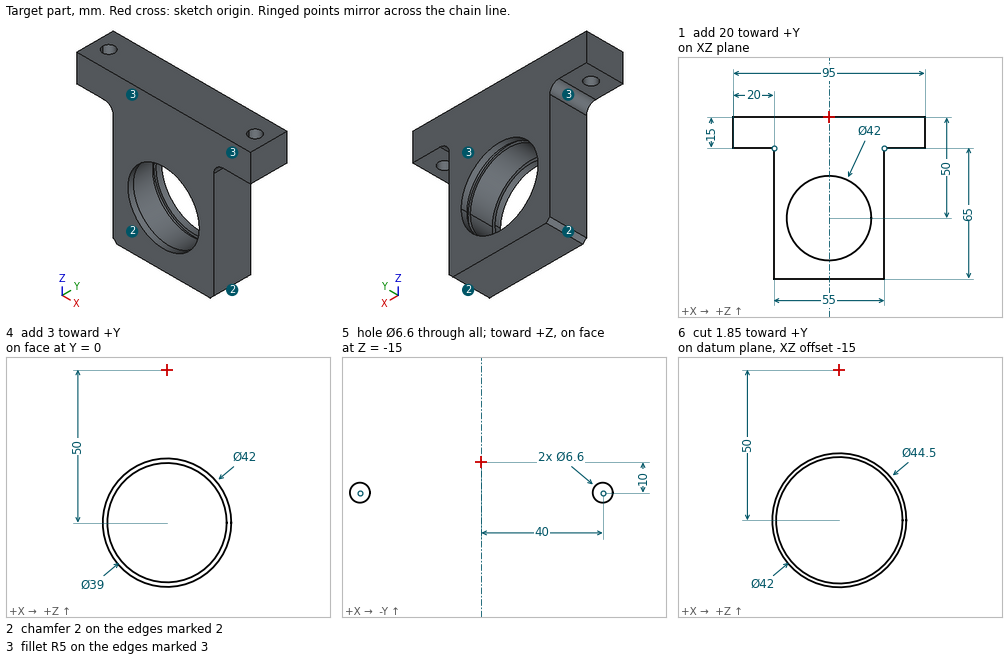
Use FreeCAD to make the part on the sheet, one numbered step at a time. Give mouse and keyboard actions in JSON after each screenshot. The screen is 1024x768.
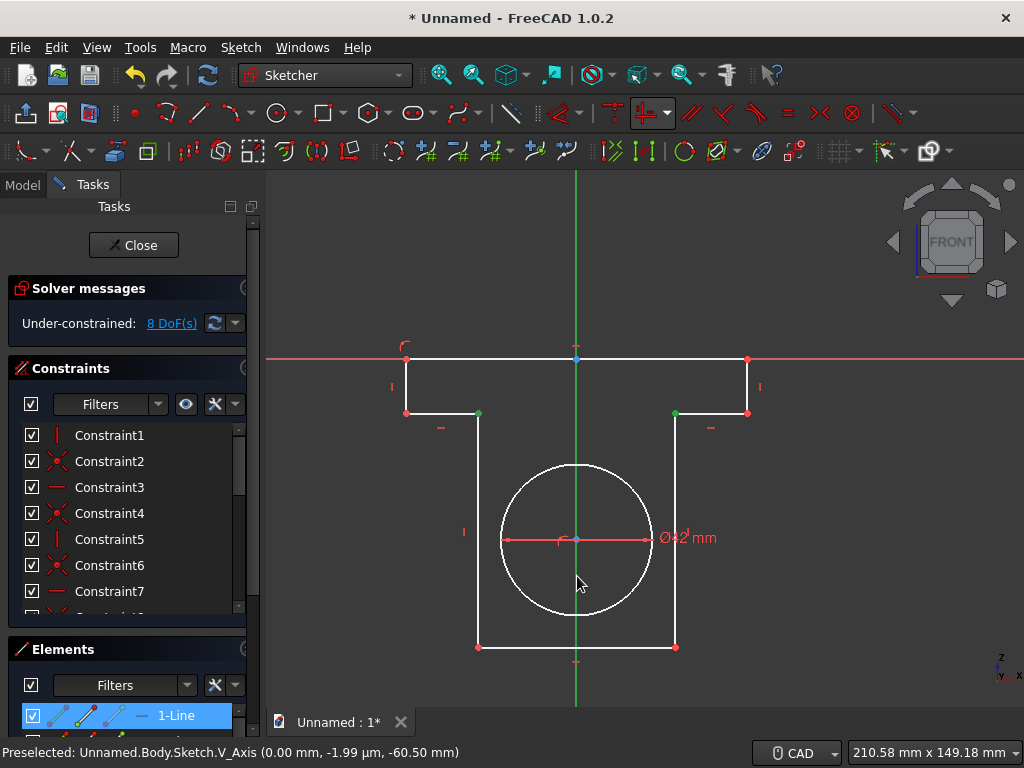
{"action": "left_click", "coordinate": [820, 114]}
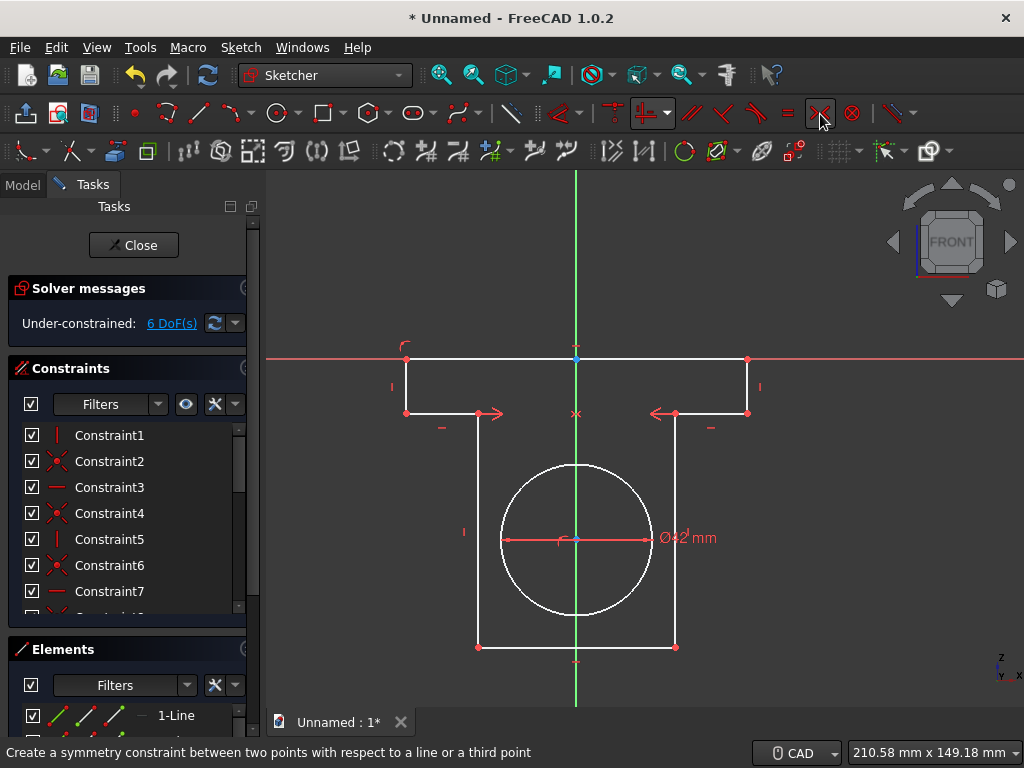
{"action": "left_click", "coordinate": [675, 484]}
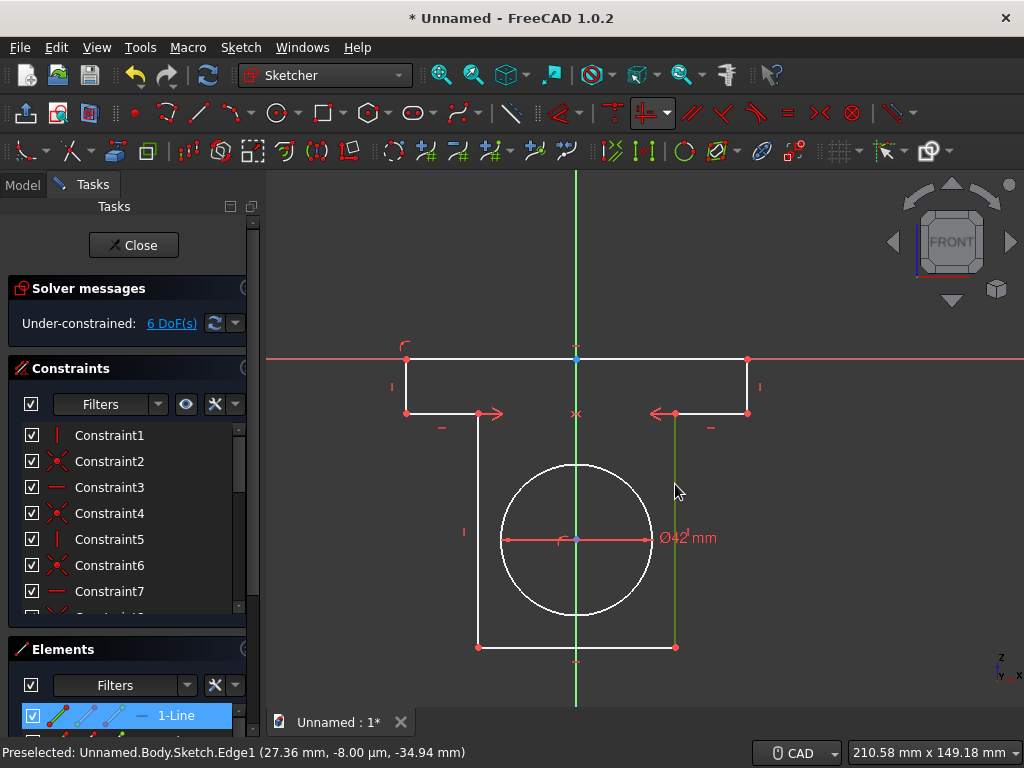
{"action": "key", "text": "i"}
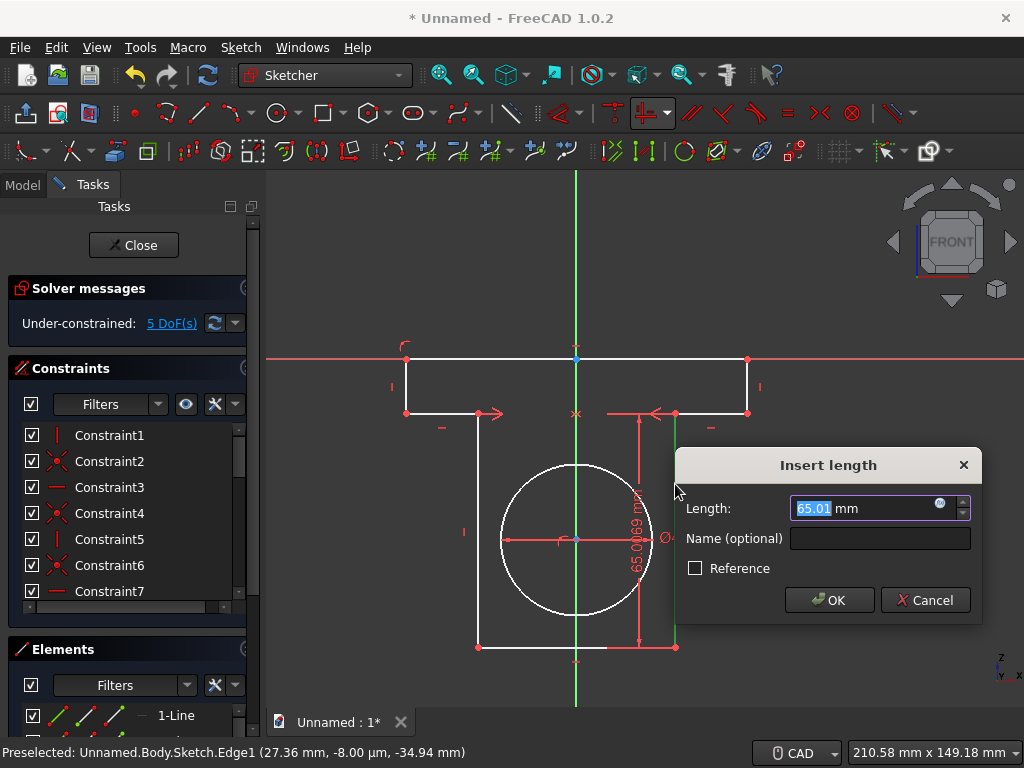
{"action": "type", "text": "65"}
{"action": "key", "text": "Return"}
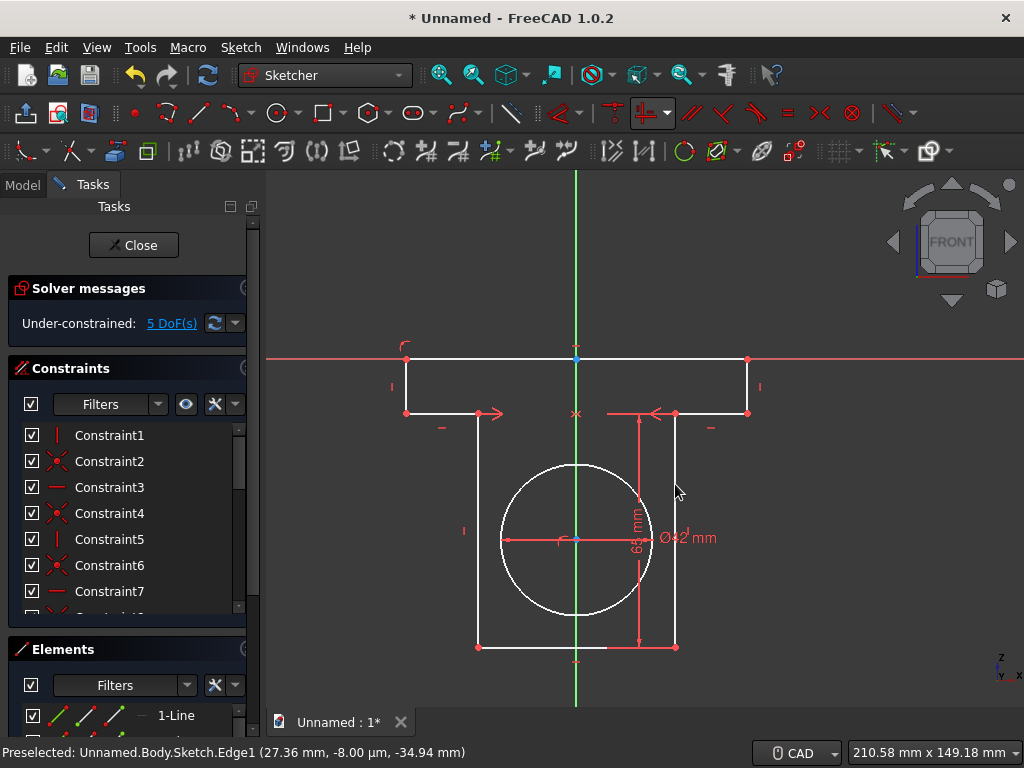
{"action": "left_click", "coordinate": [616, 648]}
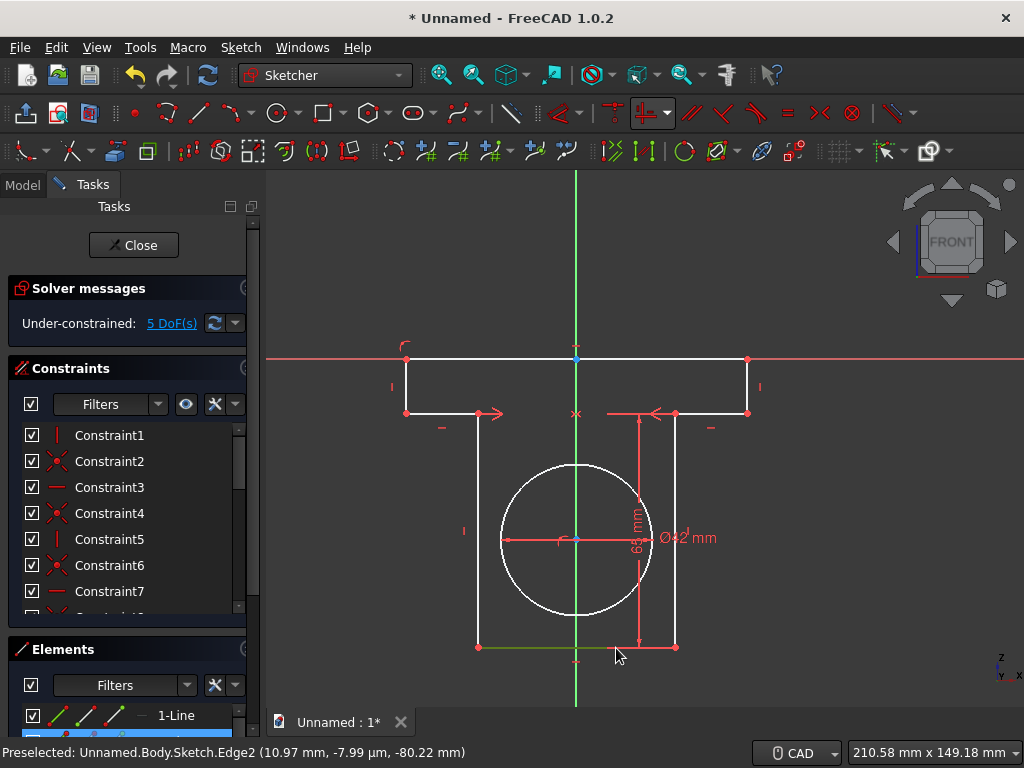
{"action": "key", "text": "l"}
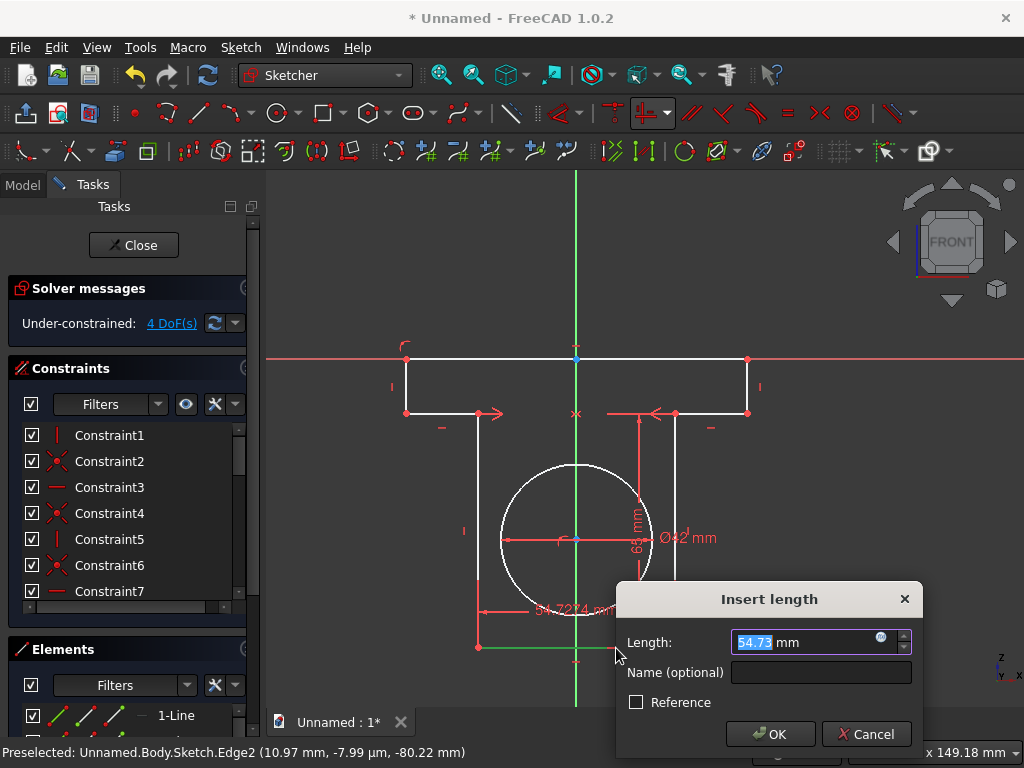
{"action": "type", "text": "55"}
{"action": "key", "text": "Return"}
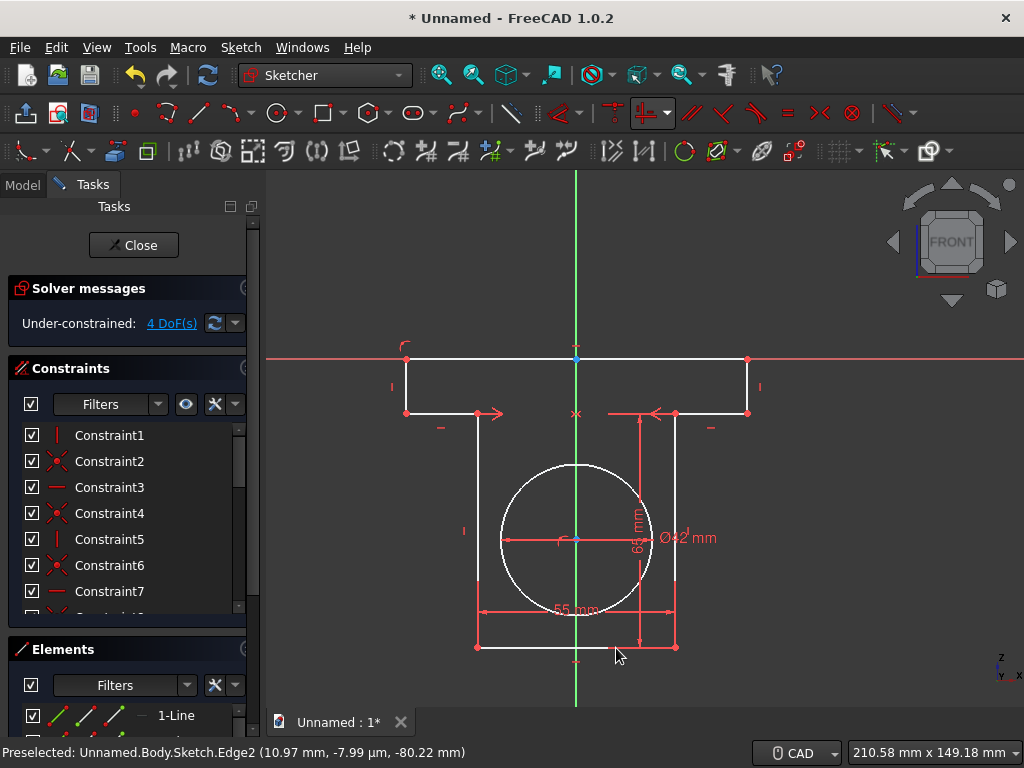
{"action": "left_click", "coordinate": [456, 414]}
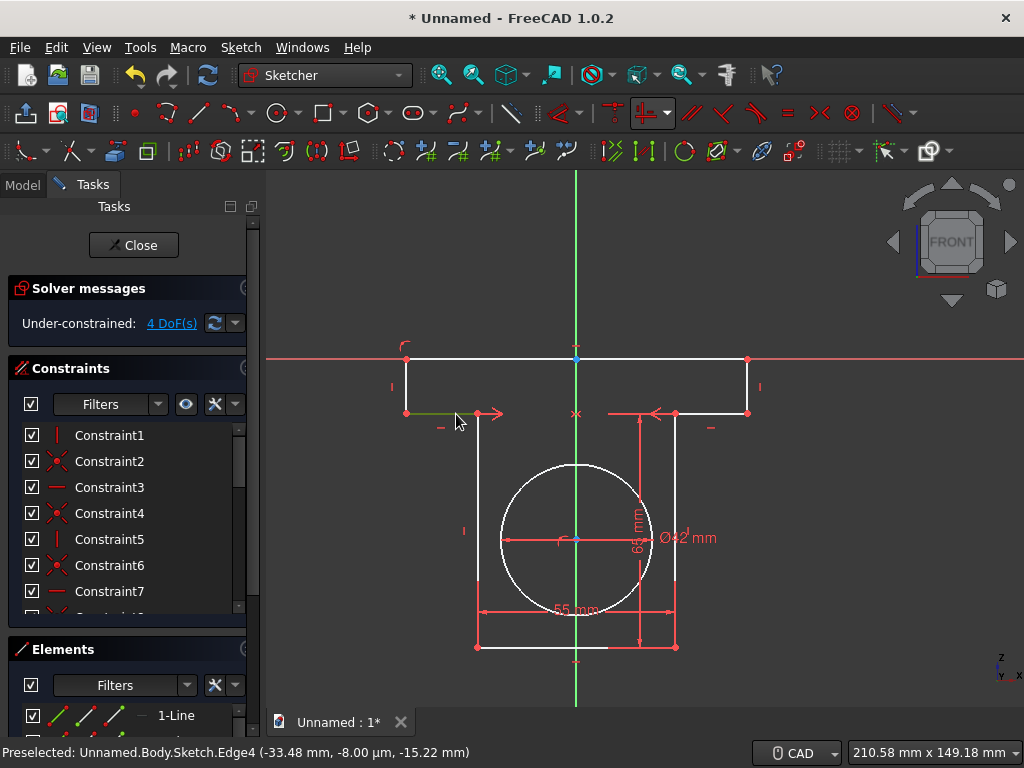
{"action": "key", "text": "l"}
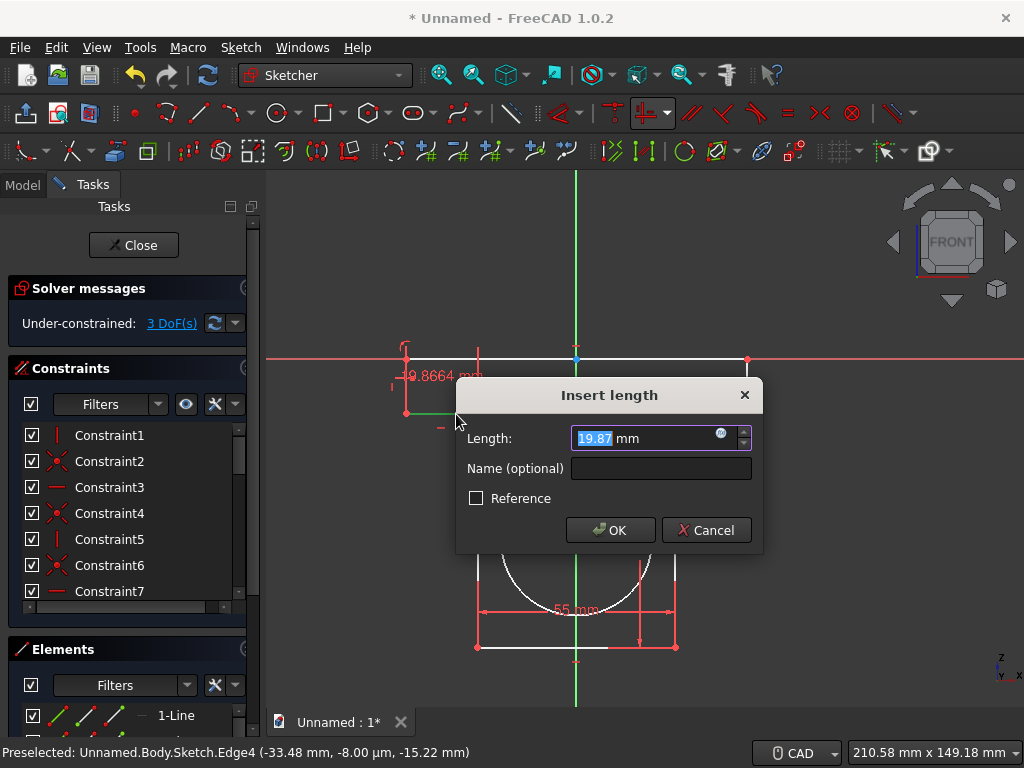
{"action": "type", "text": "20"}
{"action": "key", "text": "Return"}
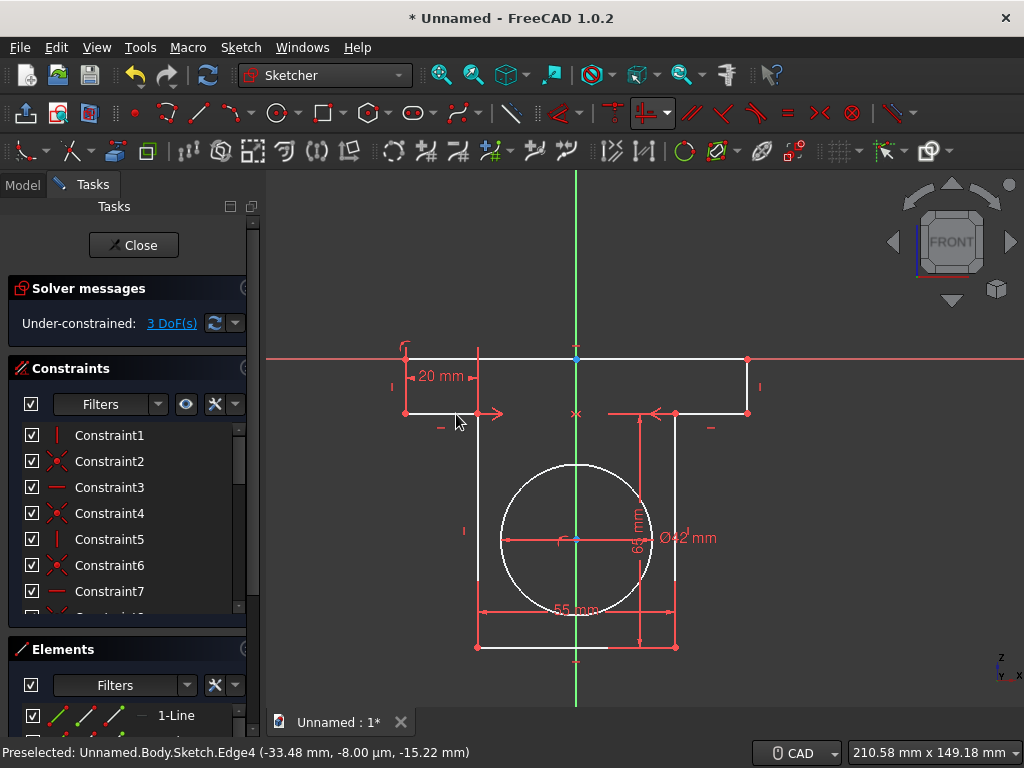
{"action": "left_click", "coordinate": [406, 398]}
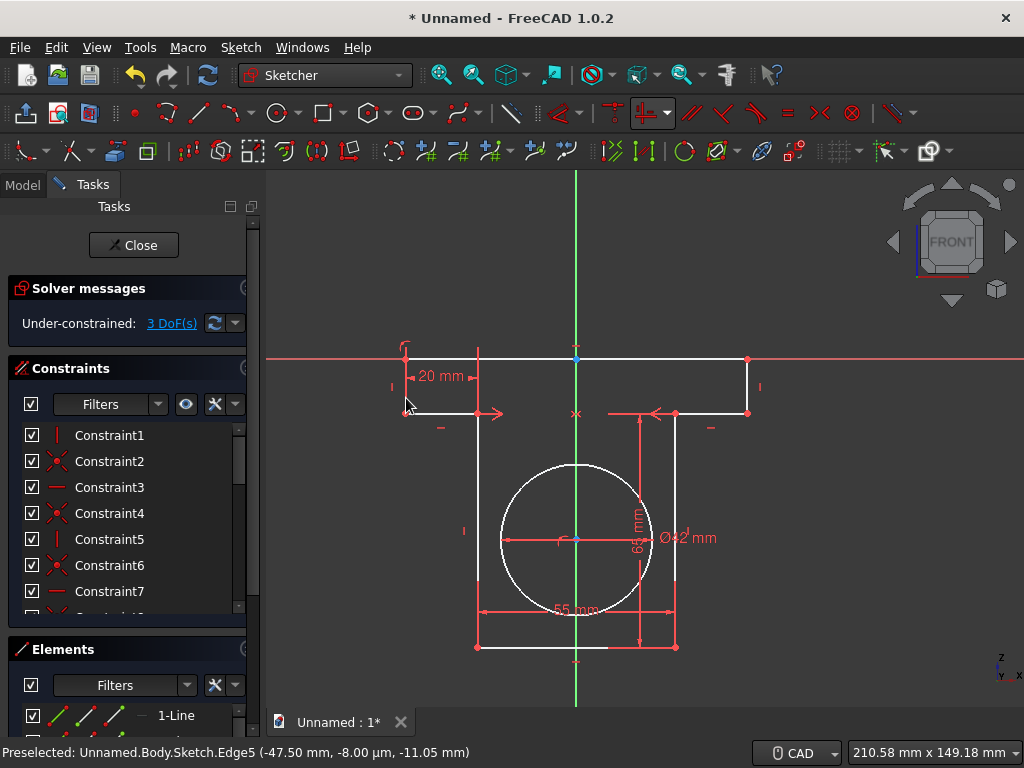
{"action": "left_click", "coordinate": [582, 114]}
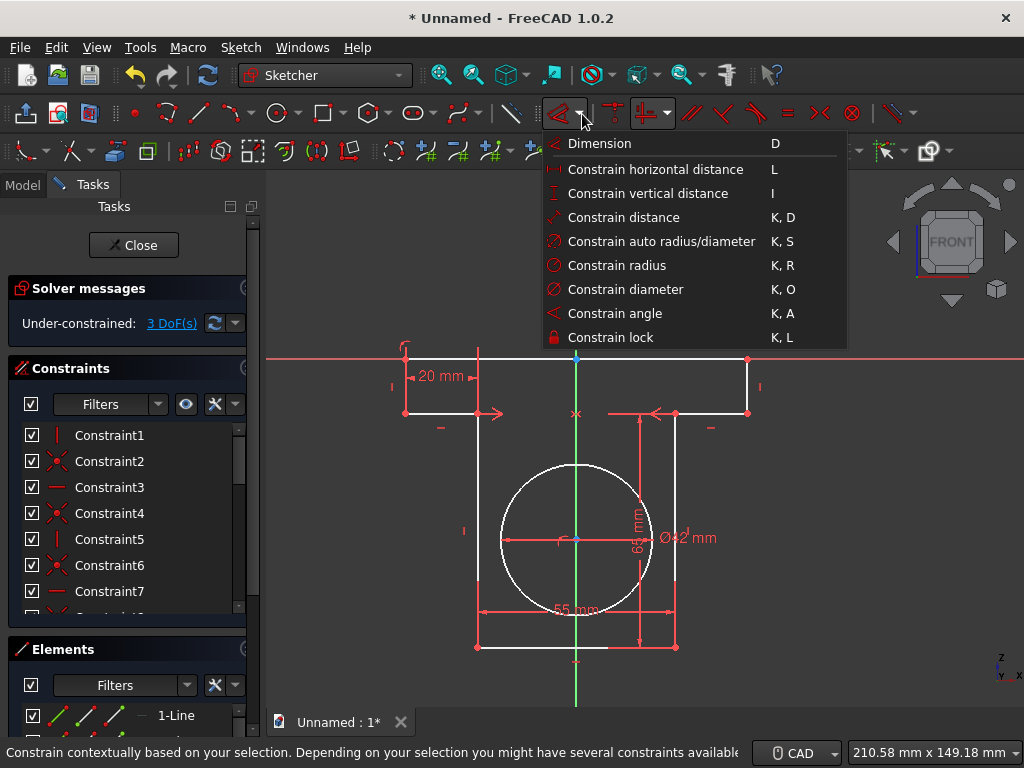
{"action": "left_click", "coordinate": [695, 193]}